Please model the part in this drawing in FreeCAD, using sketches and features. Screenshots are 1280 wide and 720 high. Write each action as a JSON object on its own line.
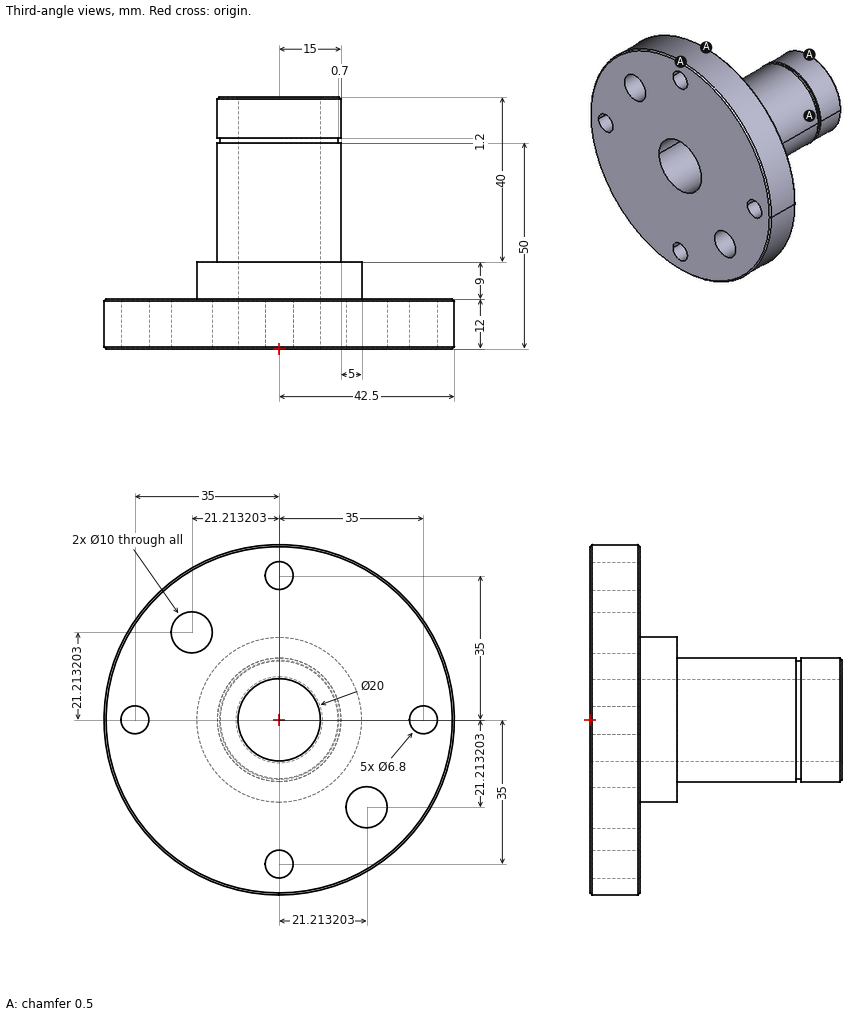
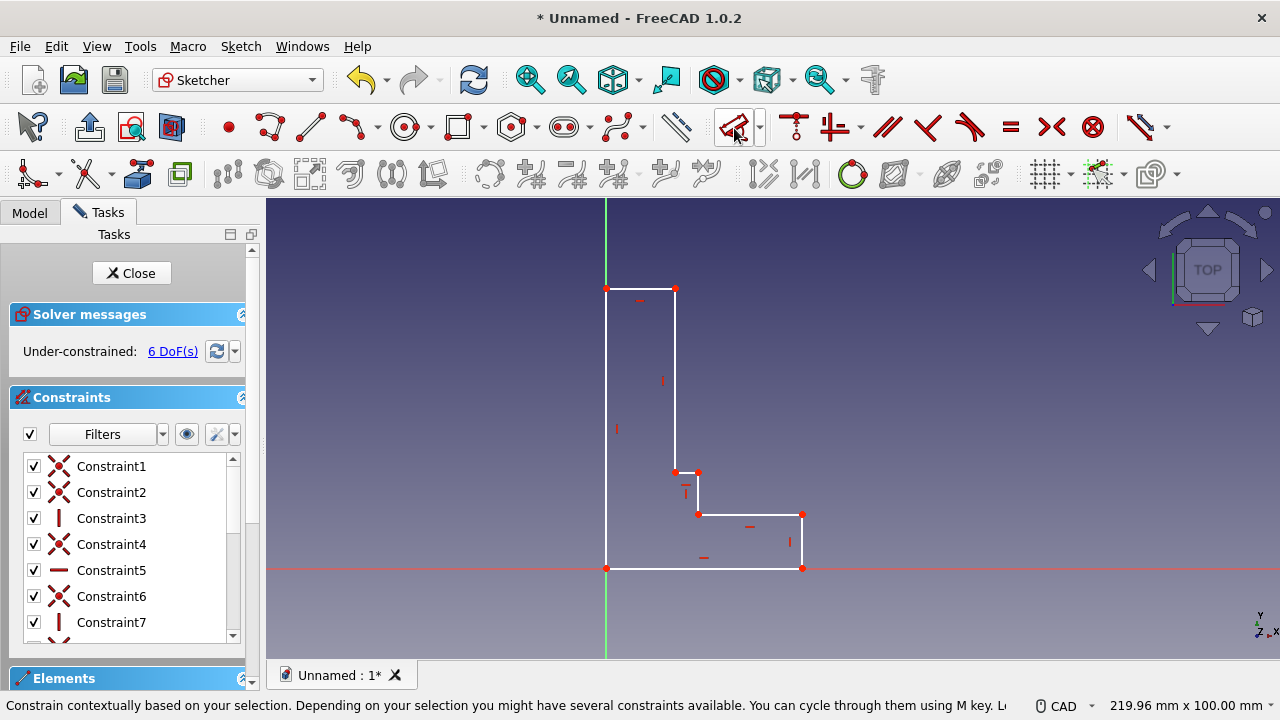
{"action": "left_click", "coordinate": [698, 502]}
{"action": "left_click", "coordinate": [664, 494]}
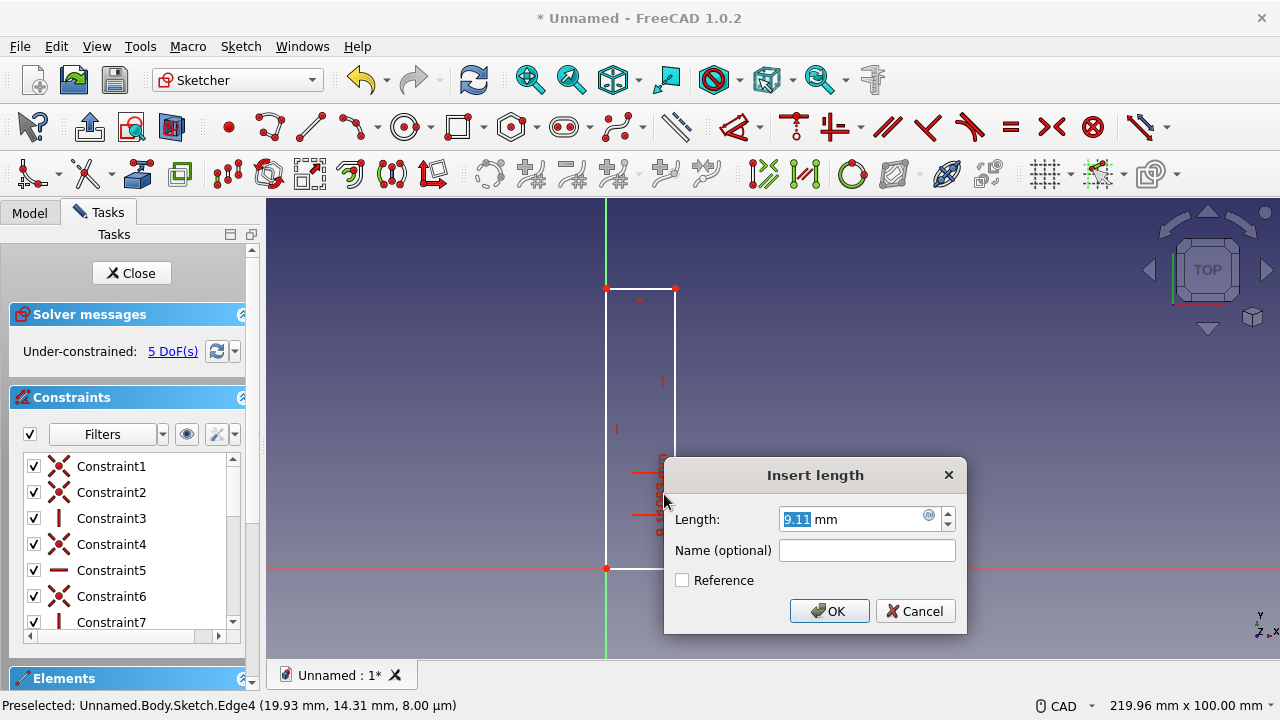
{"action": "type", "text": "9"}
{"action": "key", "text": "Return"}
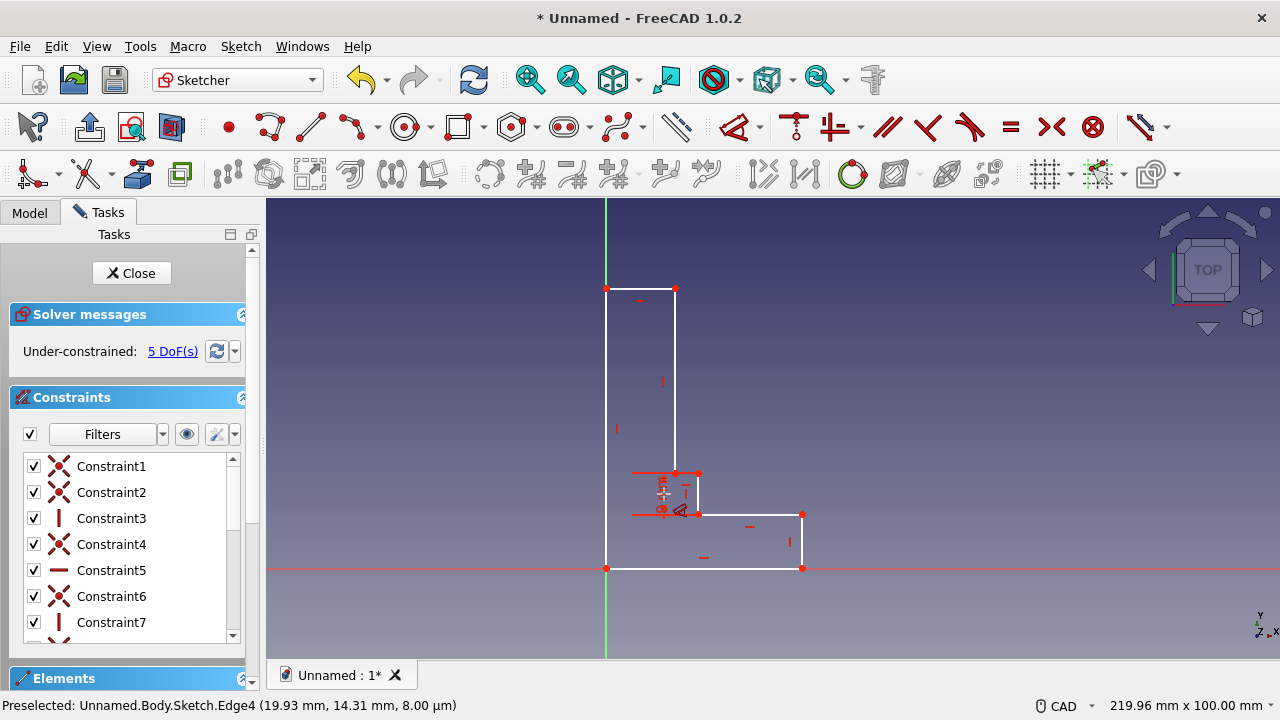
{"action": "scroll", "coordinate": [689, 473], "scroll_direction": "up", "scroll_amount": 3}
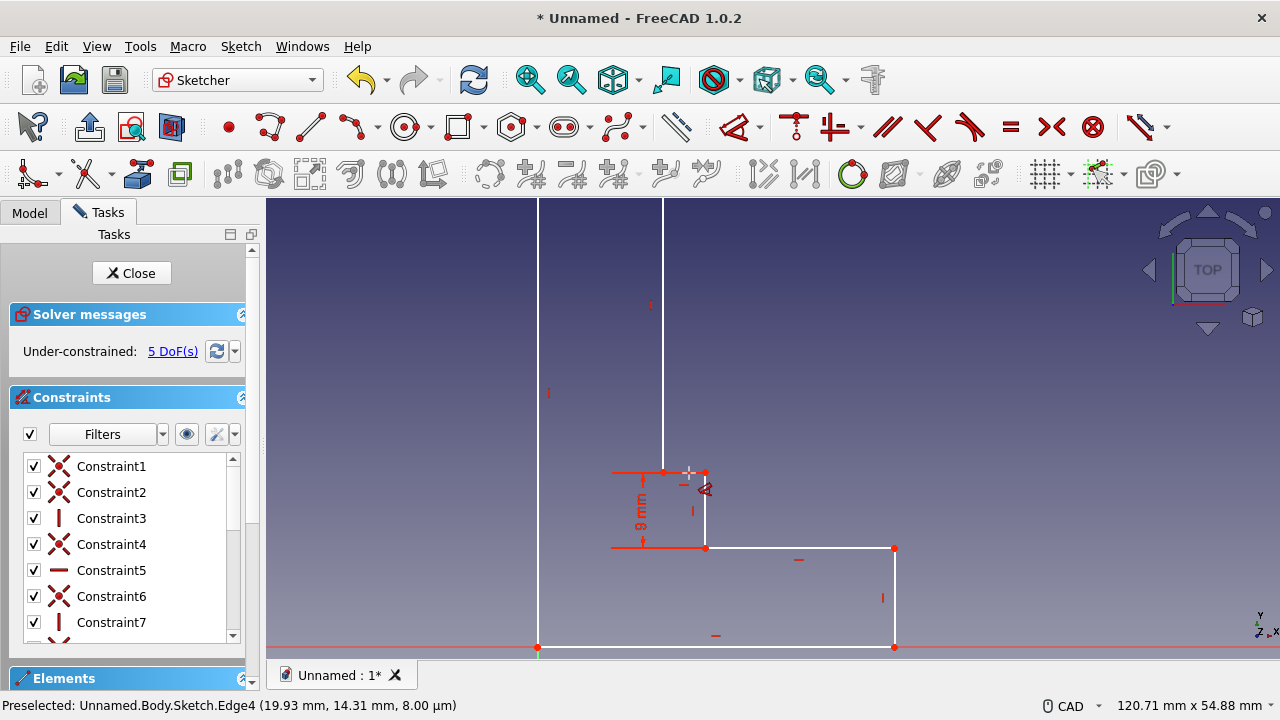
{"action": "left_click", "coordinate": [688, 473]}
{"action": "left_click", "coordinate": [684, 439]}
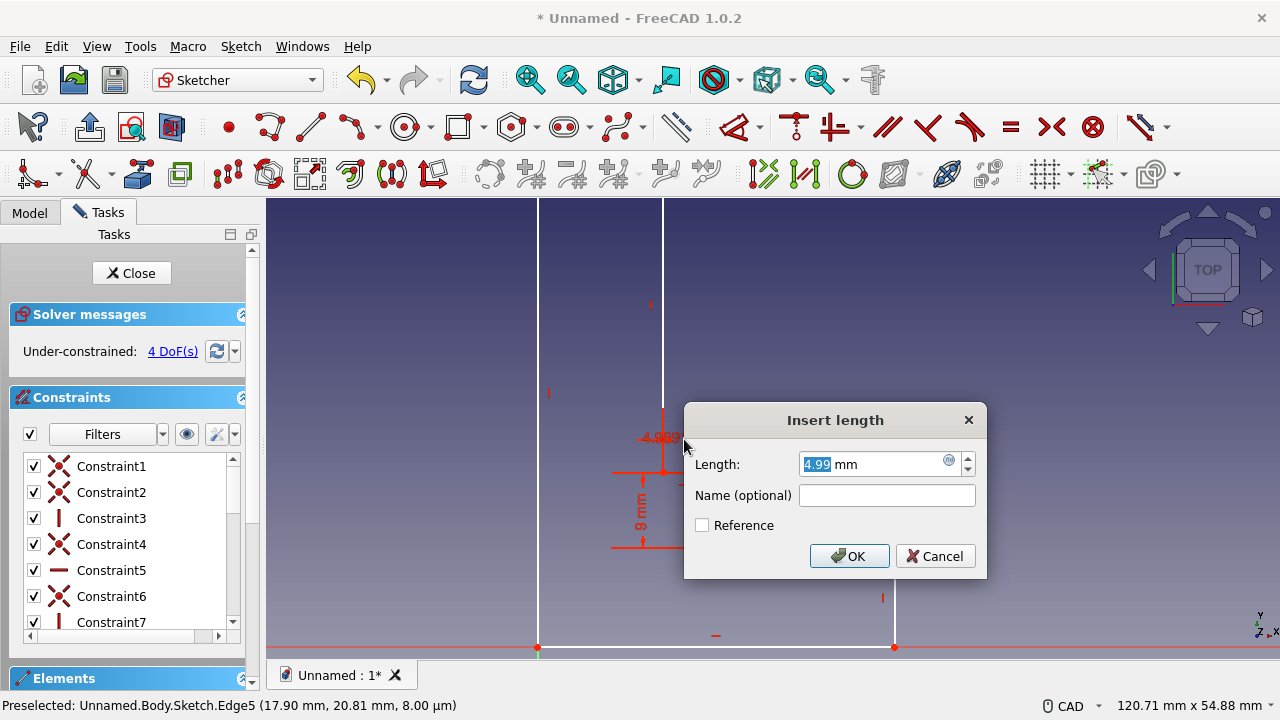
{"action": "type", "text": "5"}
{"action": "key", "text": "Return"}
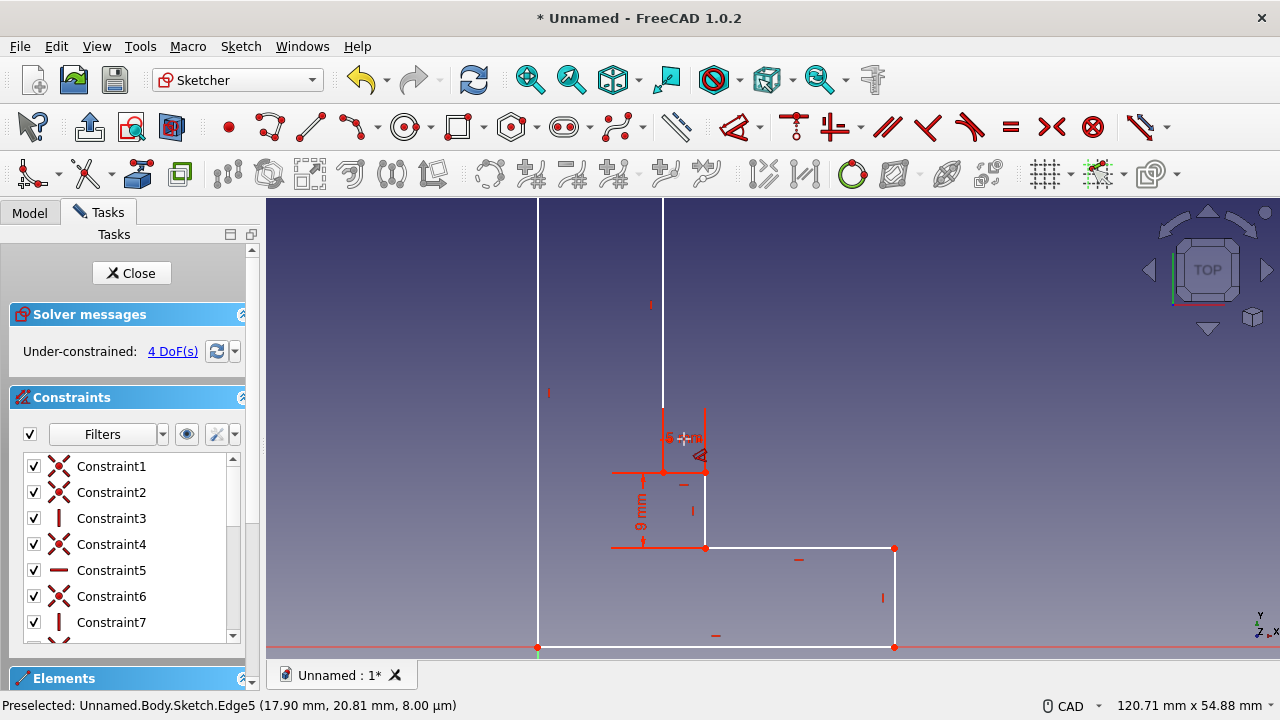
{"action": "left_click", "coordinate": [895, 618]}
{"action": "left_click", "coordinate": [929, 590]}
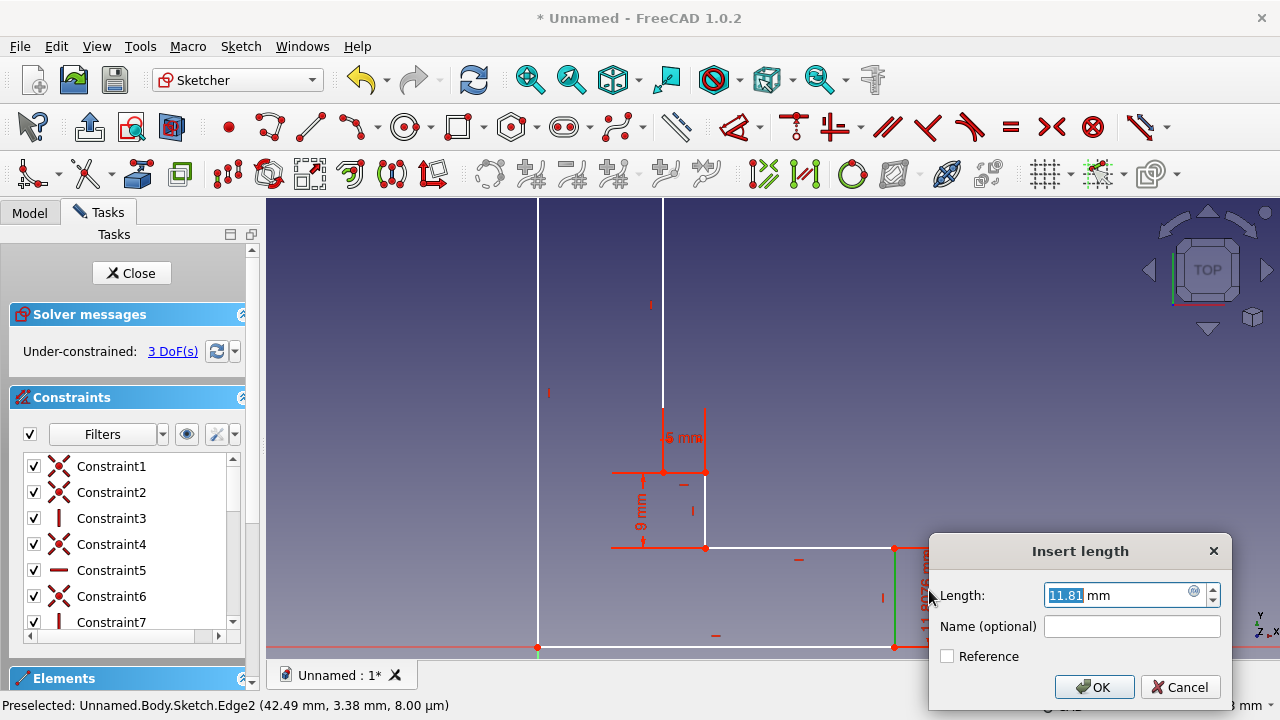
{"action": "type", "text": "12"}
{"action": "key", "text": "Return"}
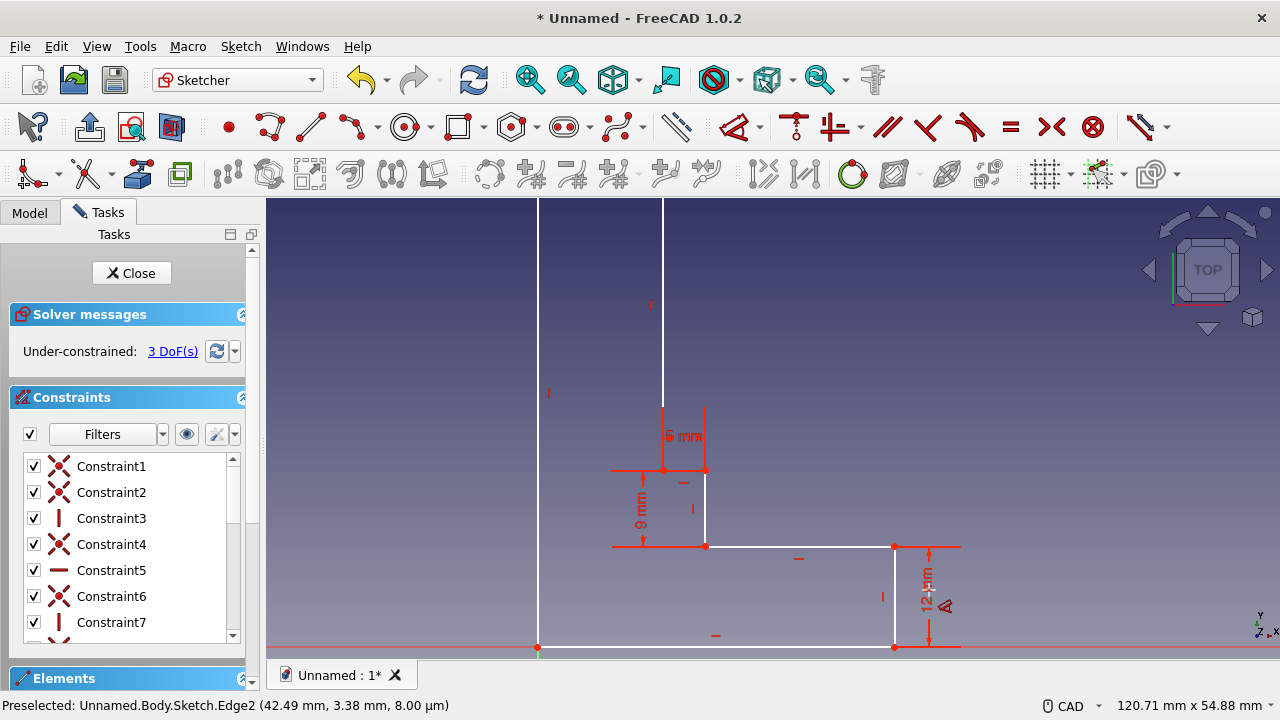
{"action": "left_click", "coordinate": [663, 371]}
{"action": "left_click", "coordinate": [629, 348]}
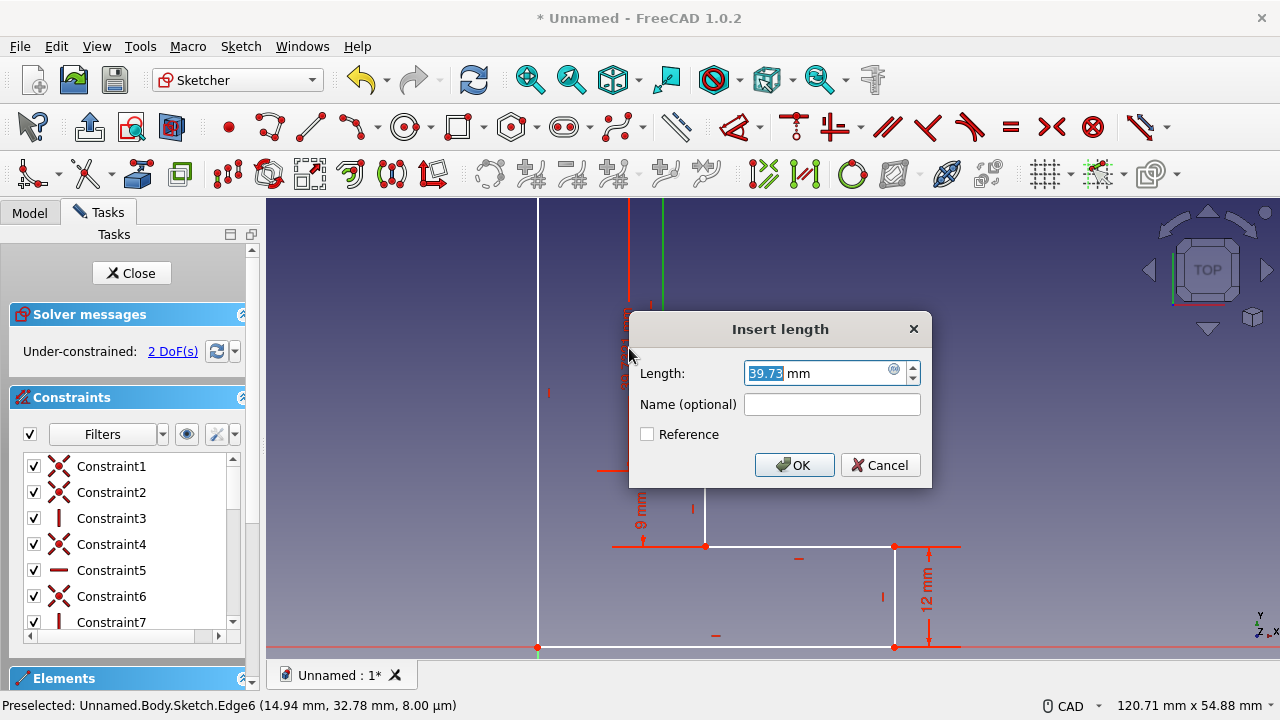
{"action": "type", "text": "40"}
{"action": "key", "text": "Return"}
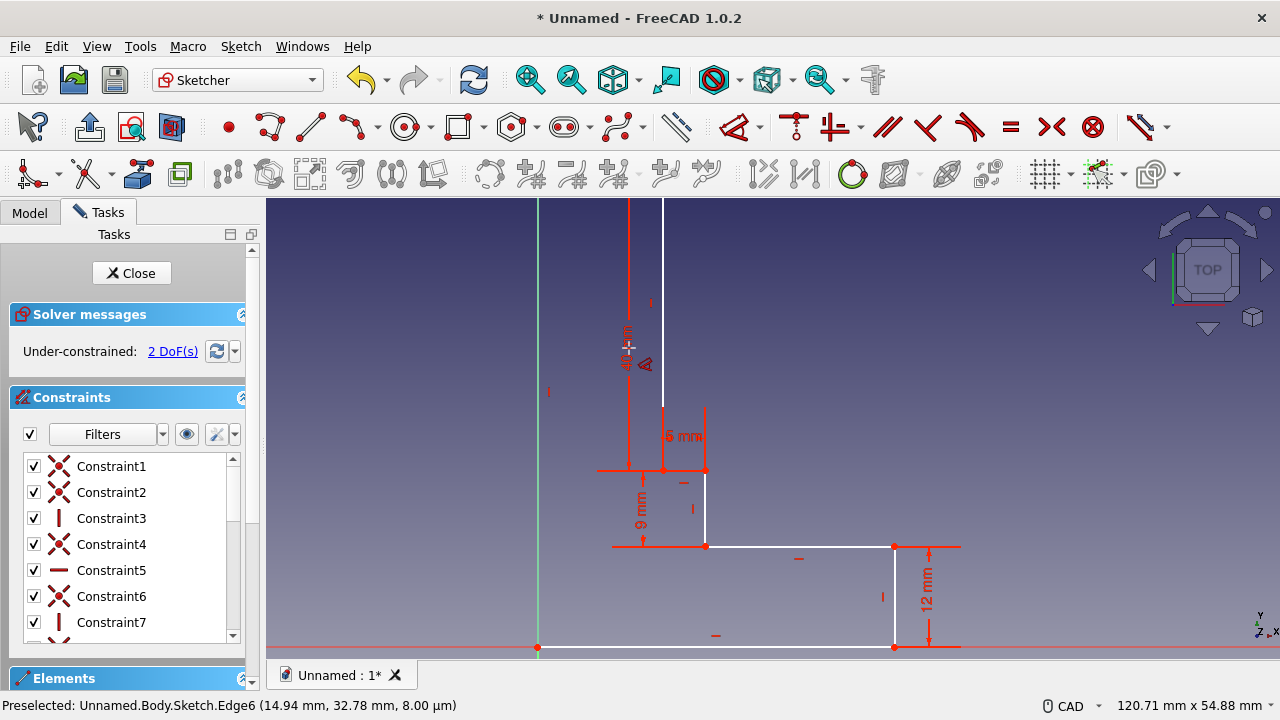
{"action": "scroll", "coordinate": [690, 474], "scroll_direction": "down", "scroll_amount": 3}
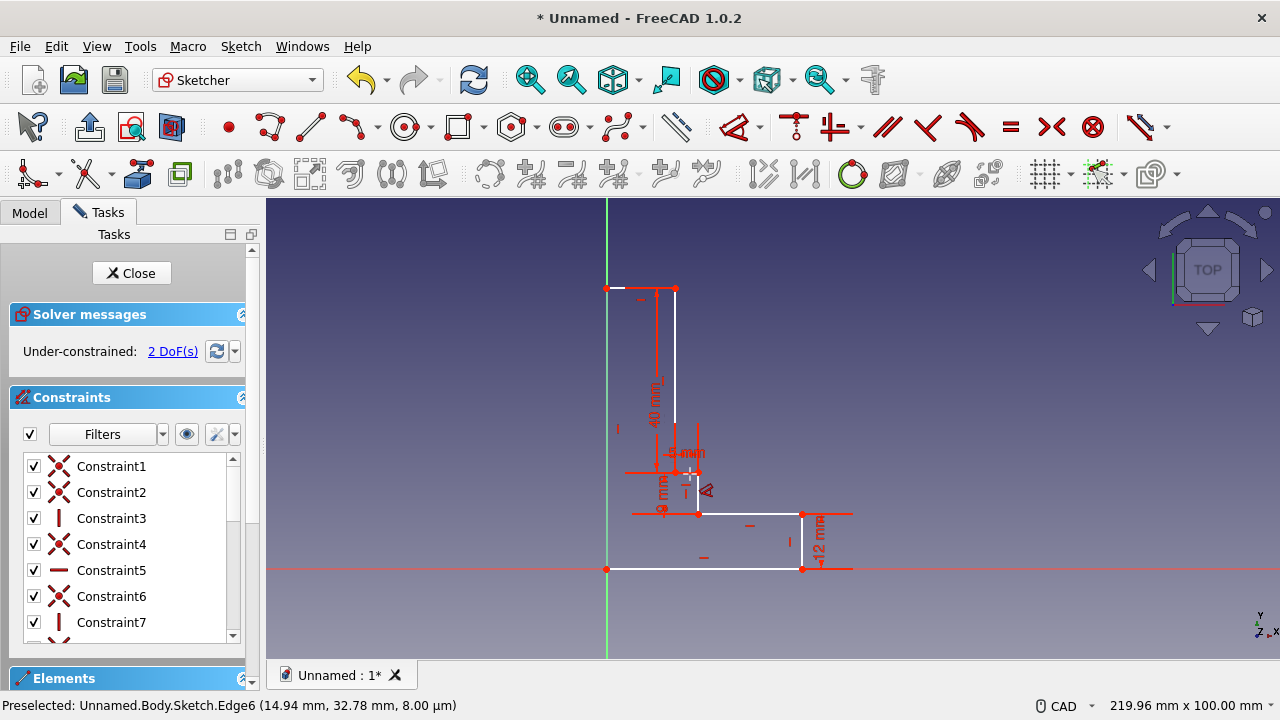
{"action": "left_click", "coordinate": [655, 288]}
{"action": "left_click", "coordinate": [641, 254]}